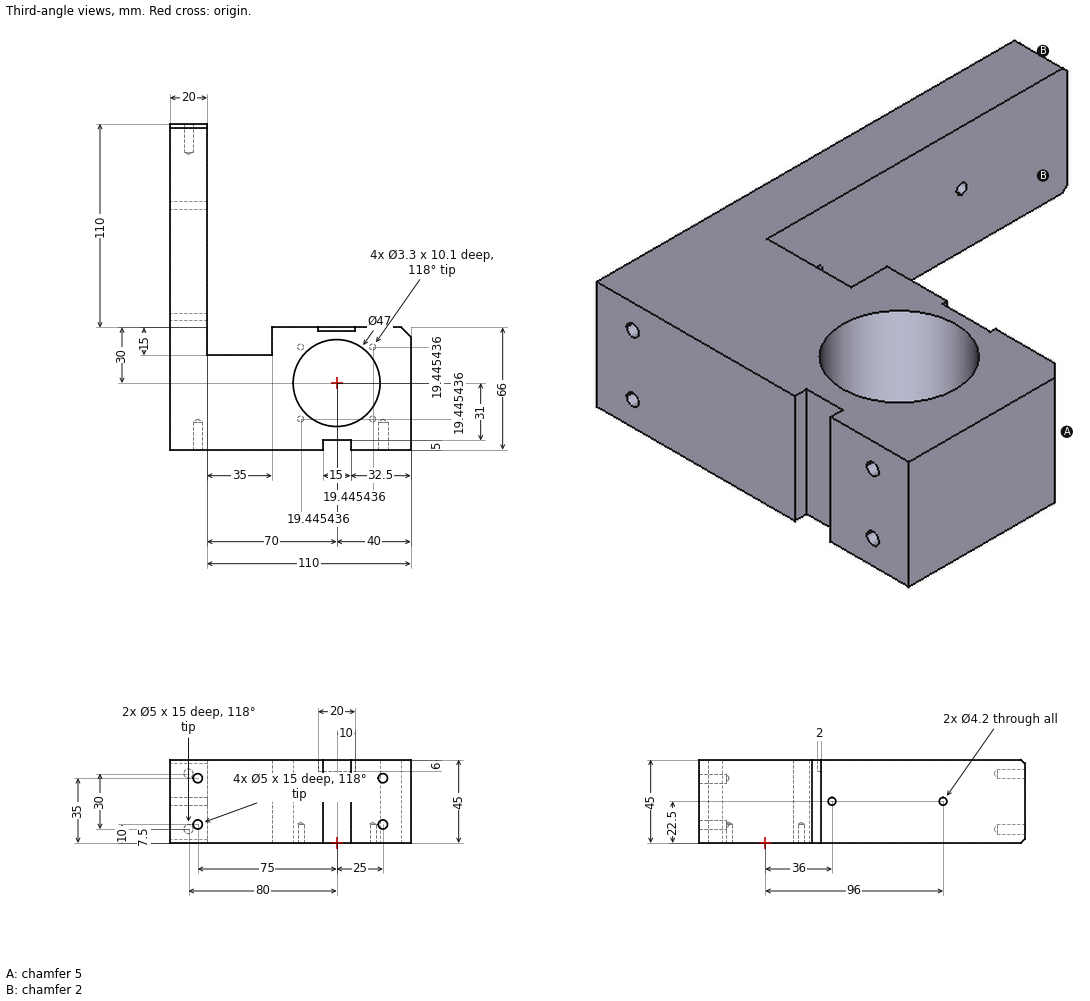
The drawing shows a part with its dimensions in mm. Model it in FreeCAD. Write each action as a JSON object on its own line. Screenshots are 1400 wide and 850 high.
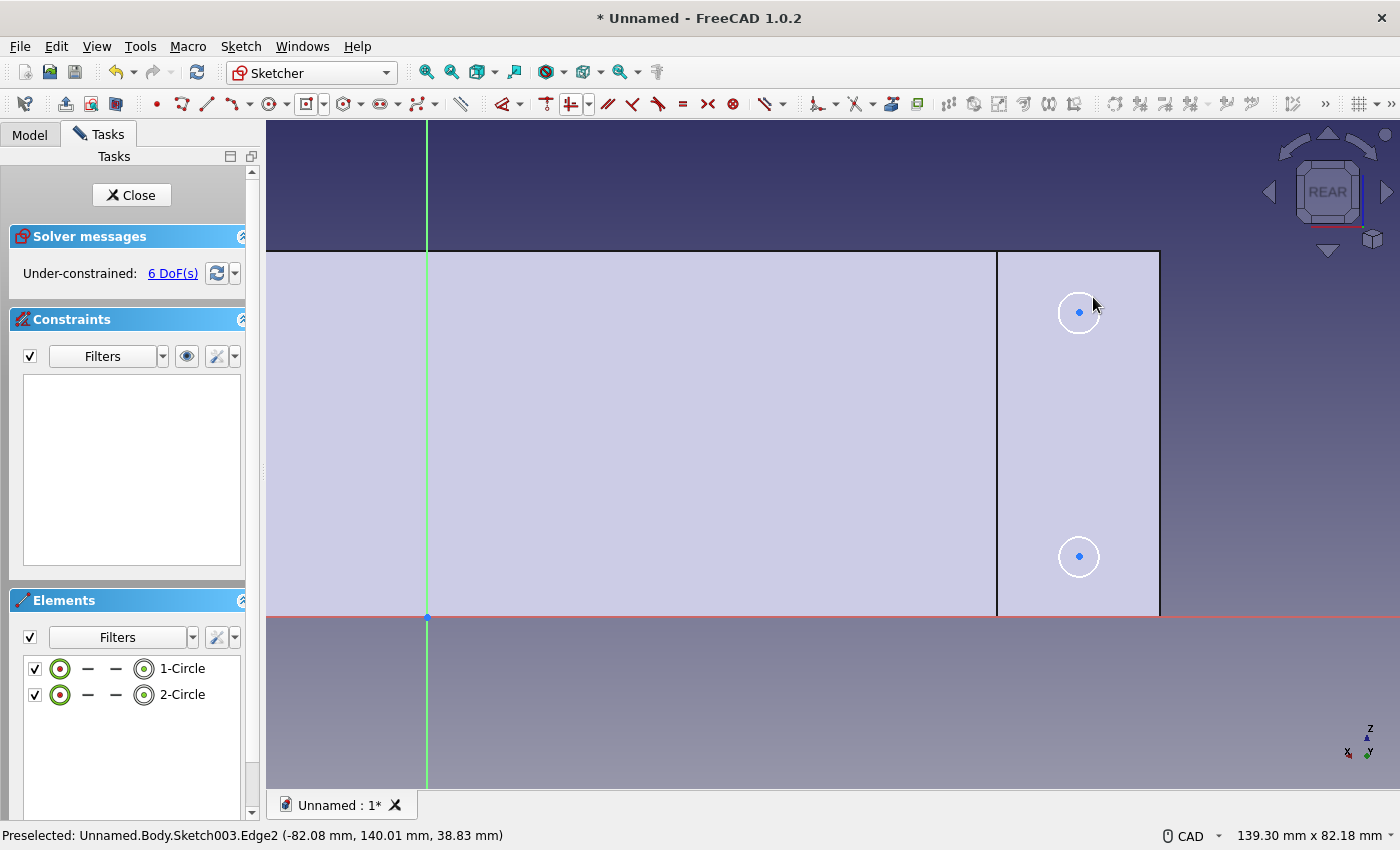
{"action": "left_click", "coordinate": [1093, 543]}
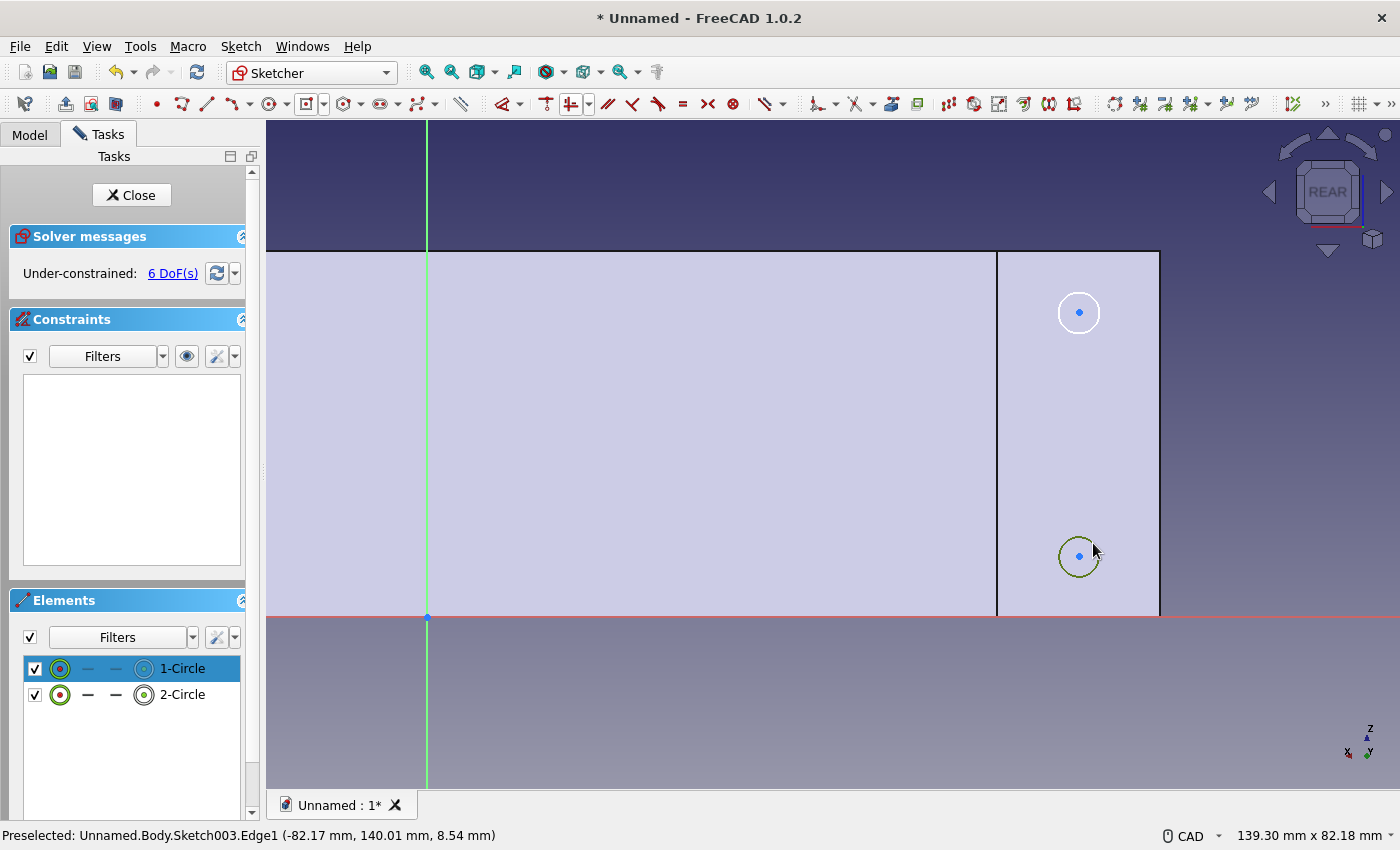
{"action": "left_click", "coordinate": [1093, 298]}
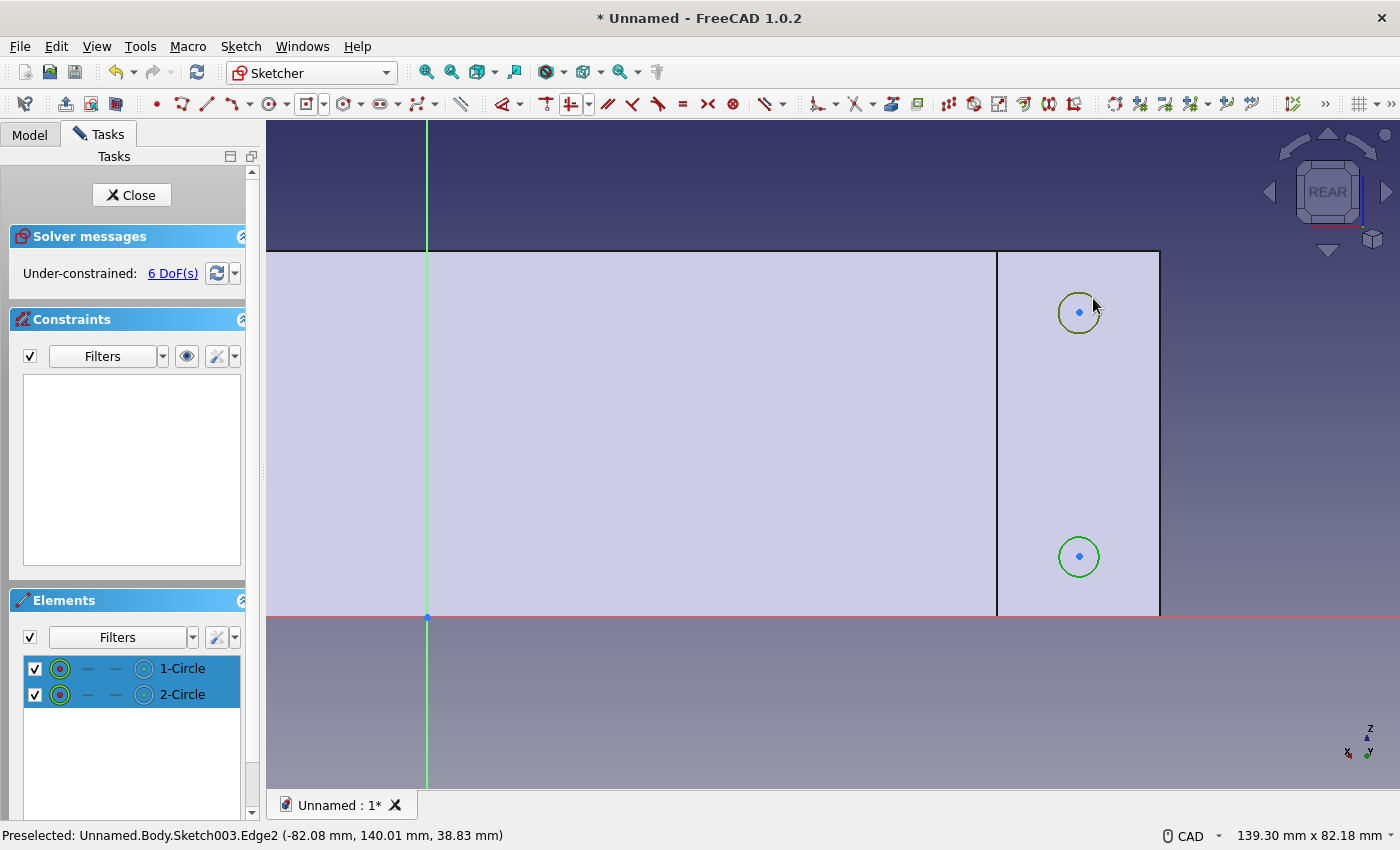
{"action": "left_click", "coordinate": [683, 104]}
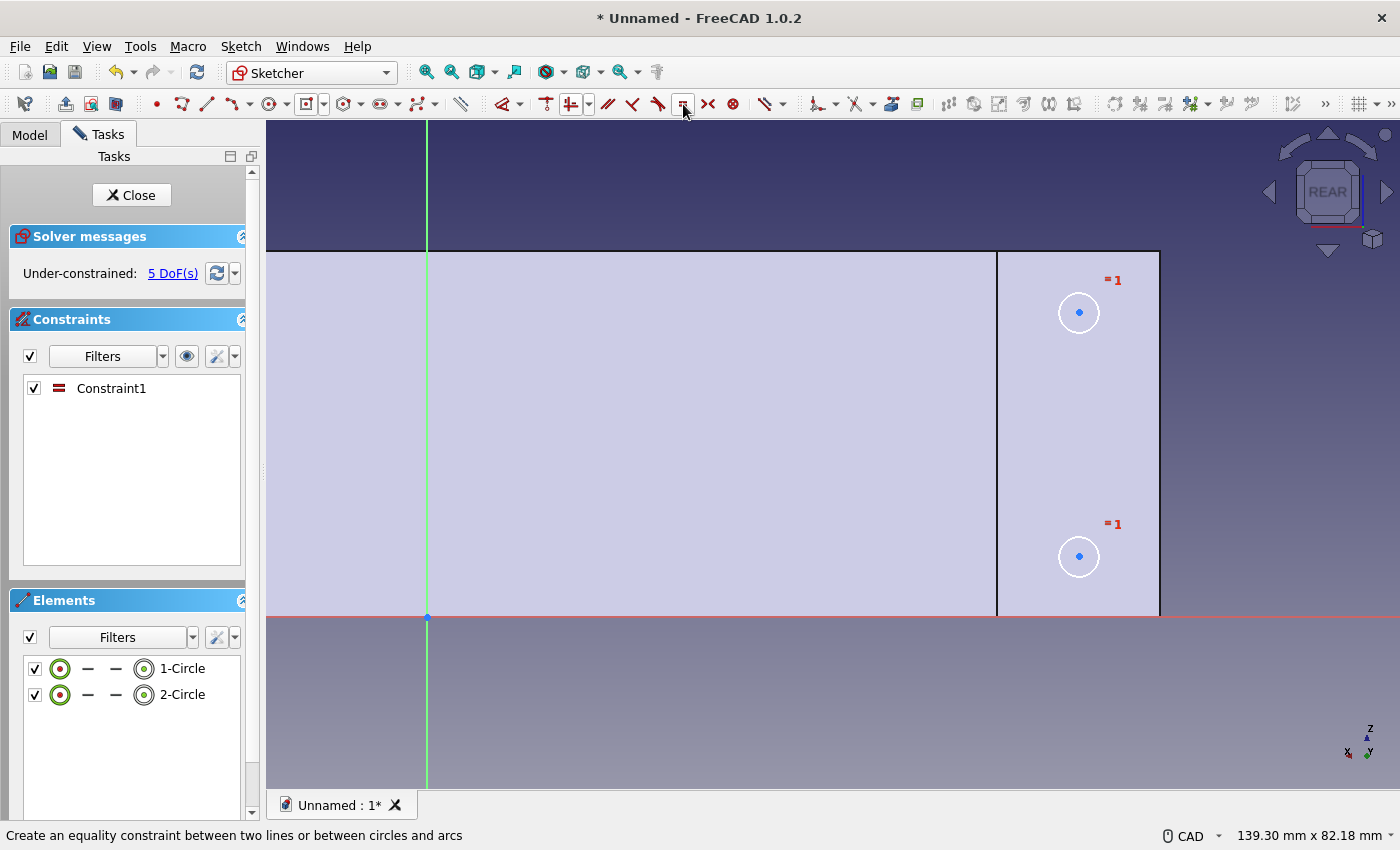
{"action": "left_click", "coordinate": [1079, 557]}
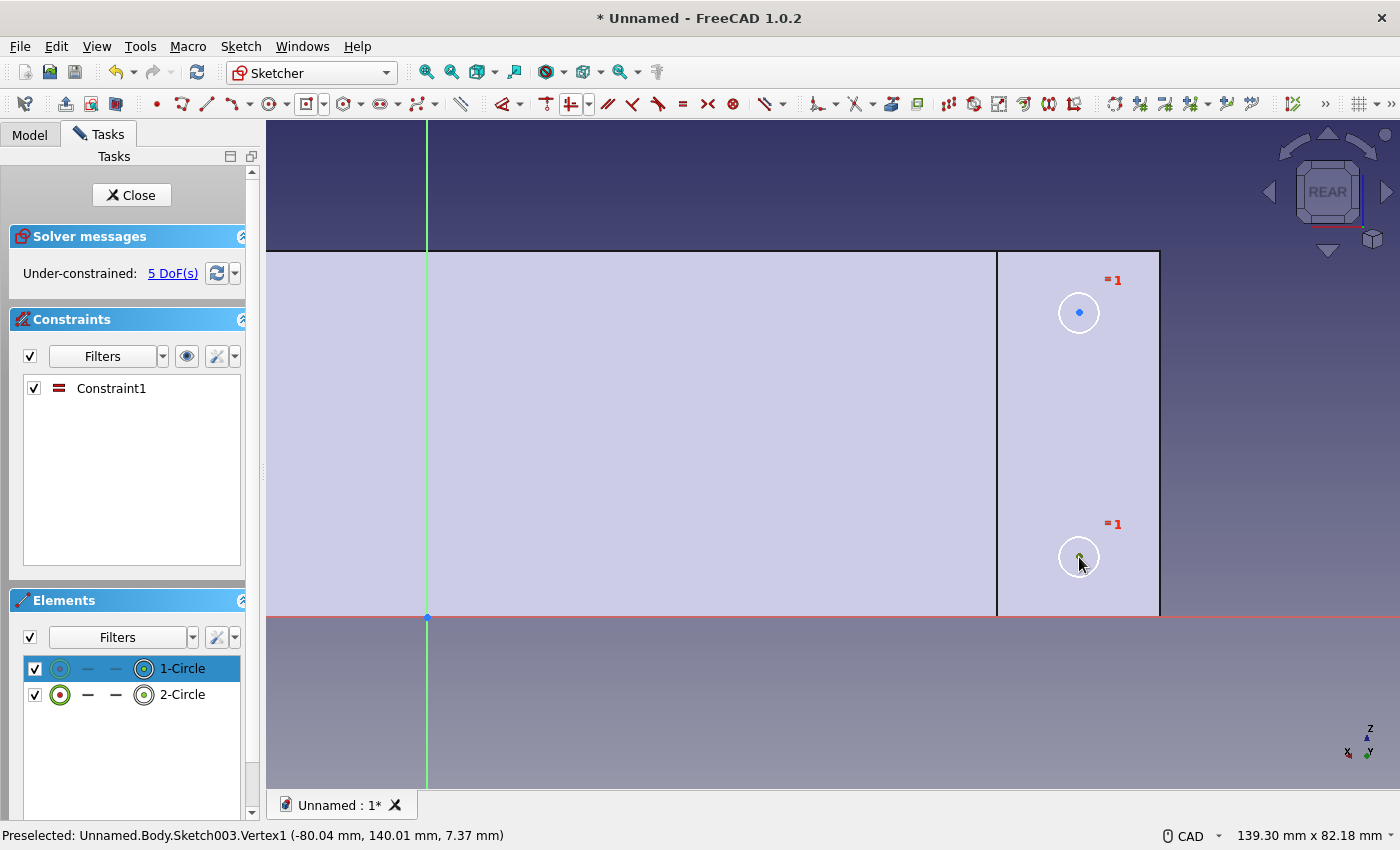
{"action": "left_click", "coordinate": [1079, 313]}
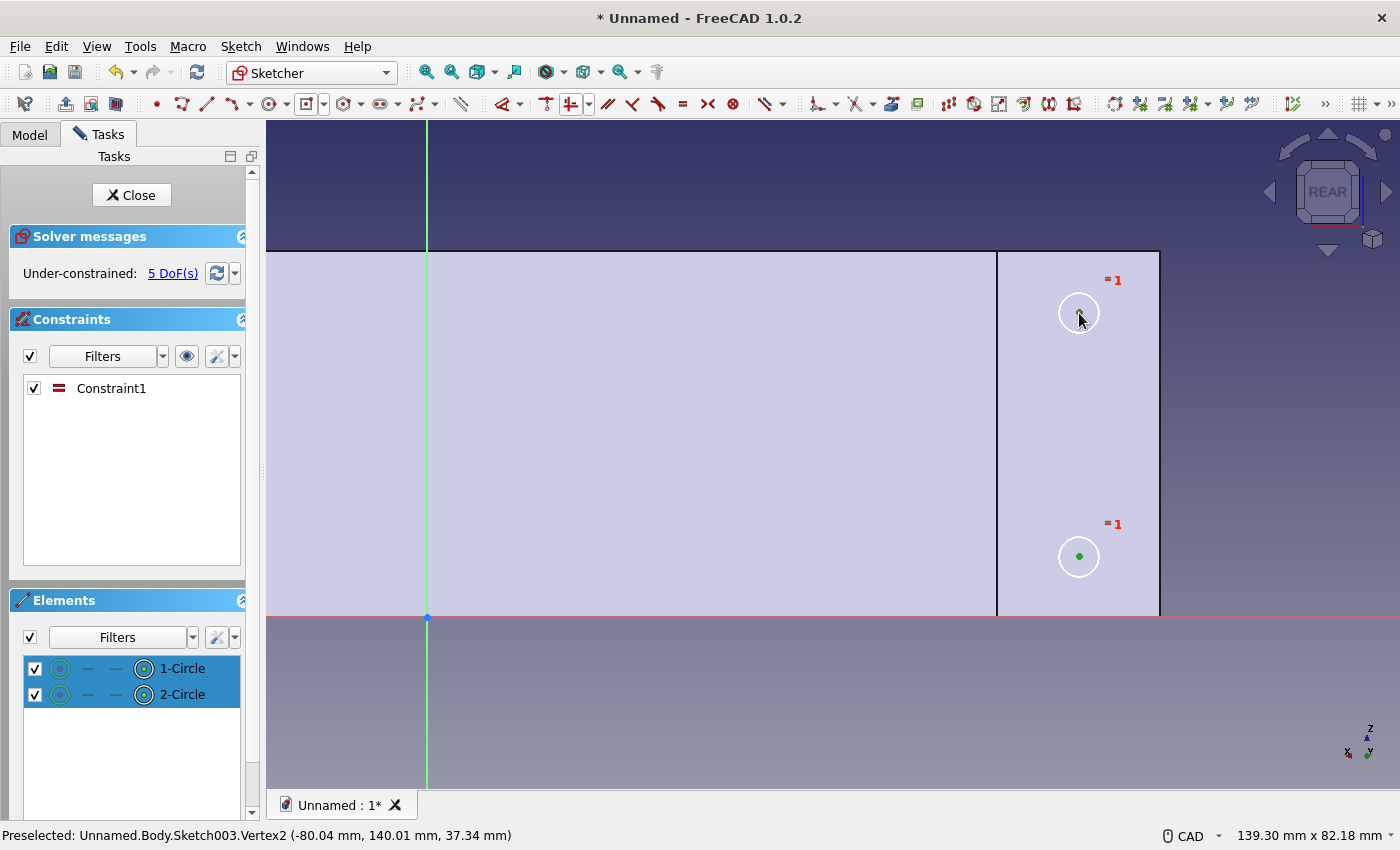
{"action": "left_click", "coordinate": [588, 104]}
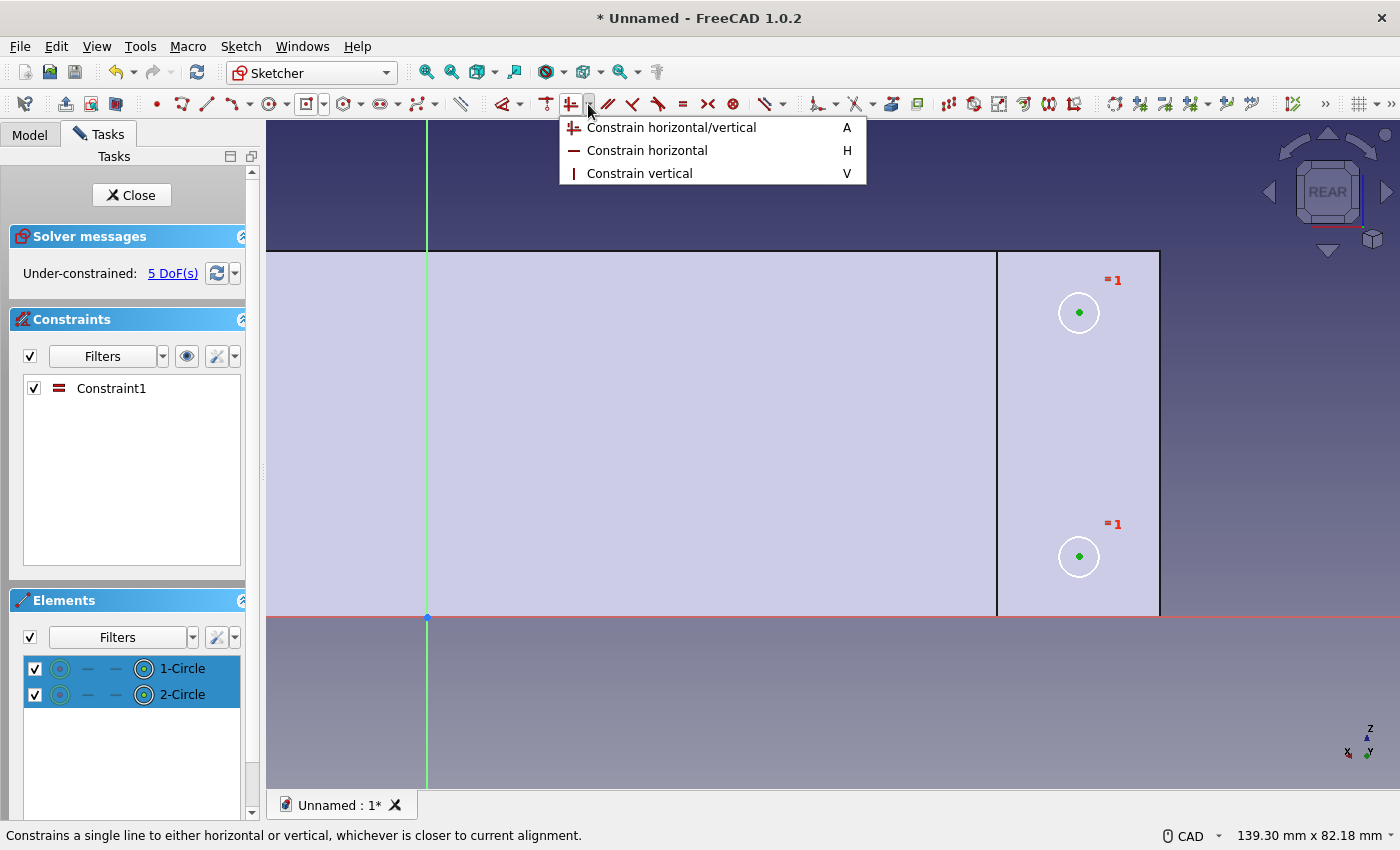
{"action": "left_click", "coordinate": [713, 174]}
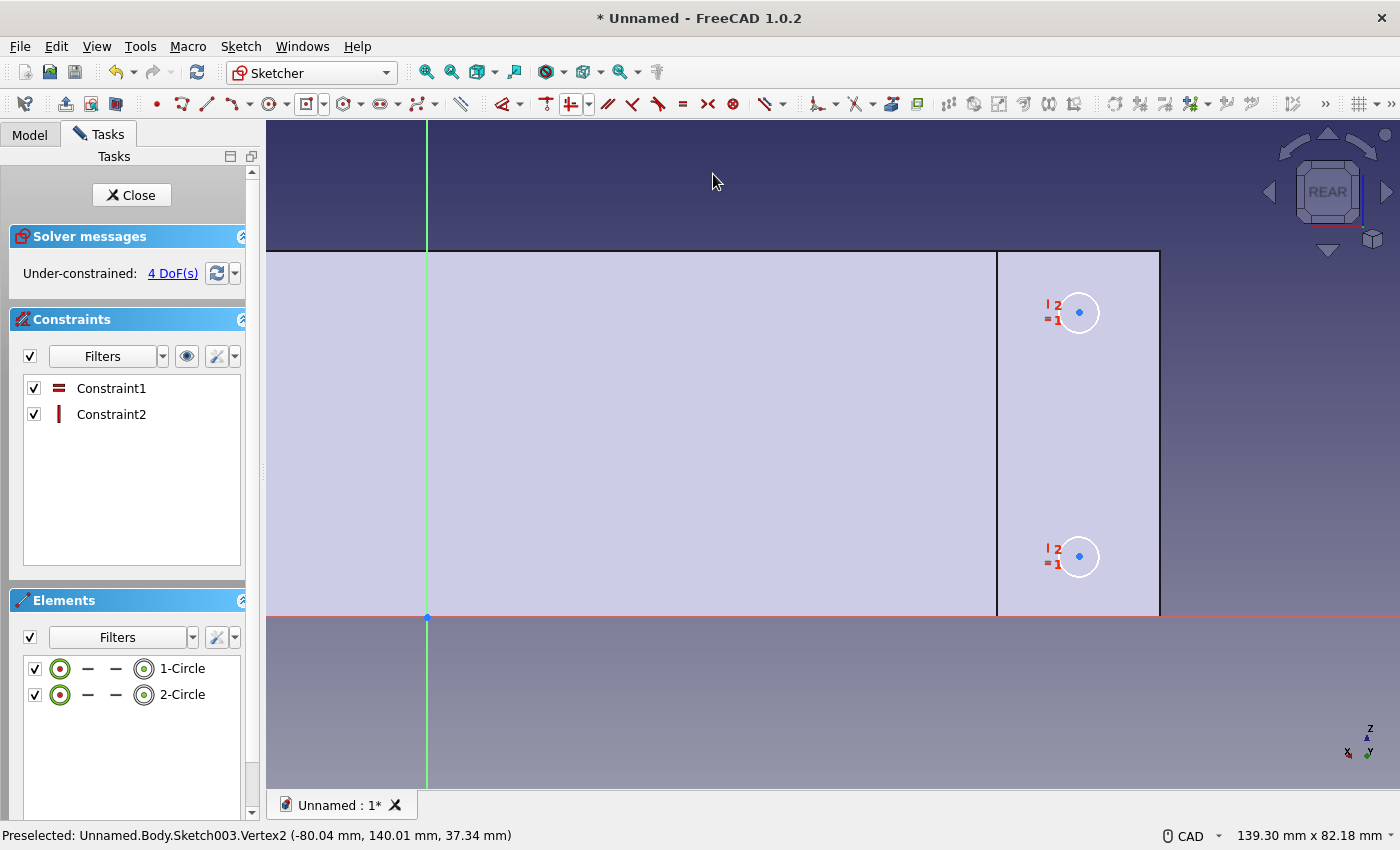
{"action": "key", "text": "d"}